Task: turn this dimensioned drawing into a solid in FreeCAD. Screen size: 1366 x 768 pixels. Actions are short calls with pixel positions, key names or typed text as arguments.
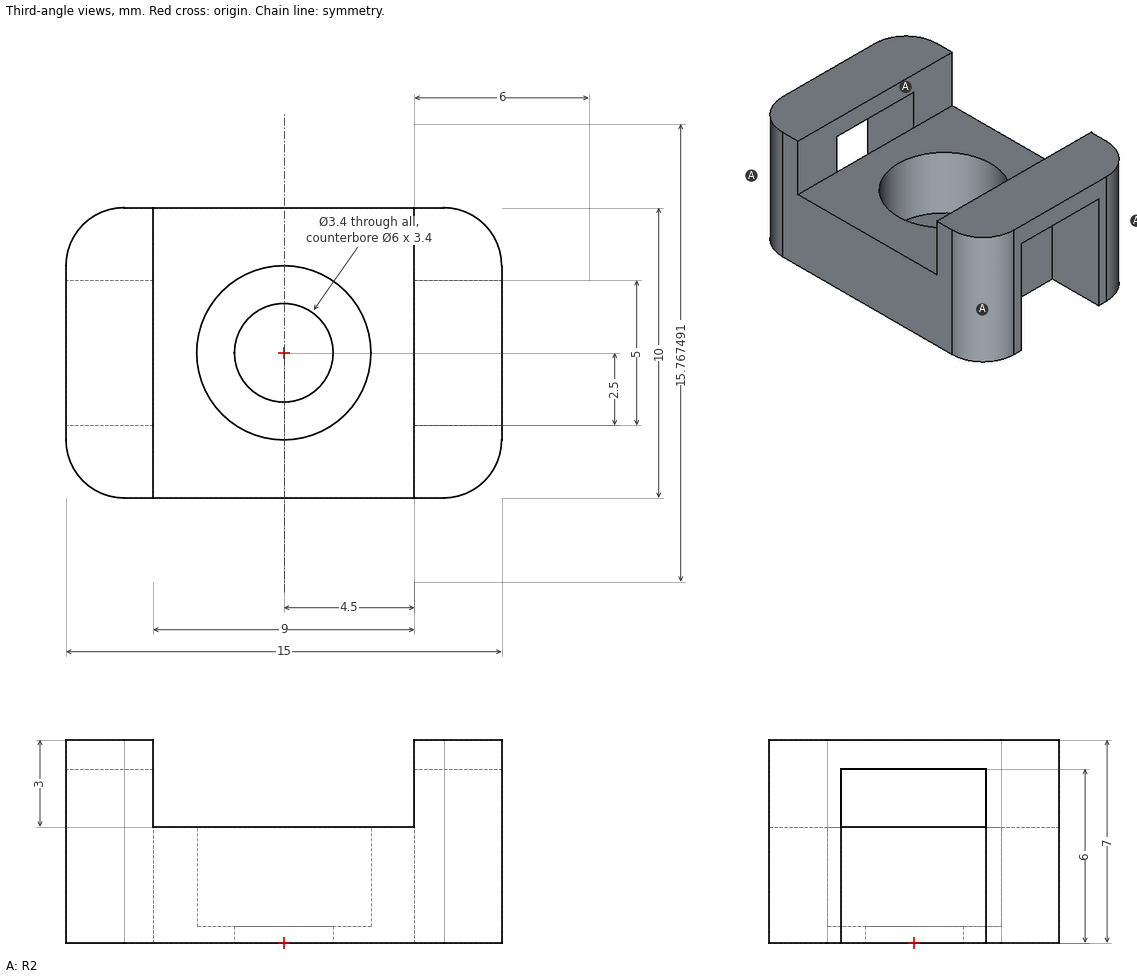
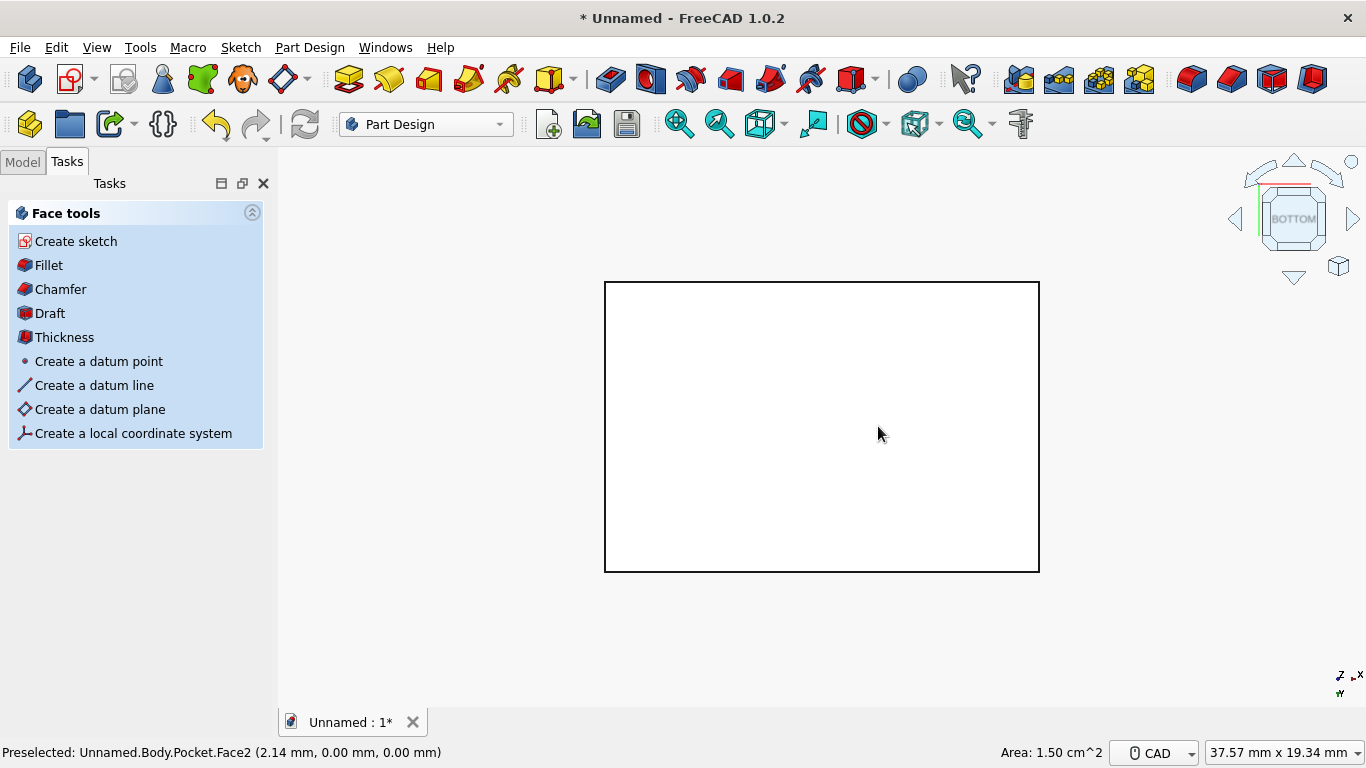
click(70, 80)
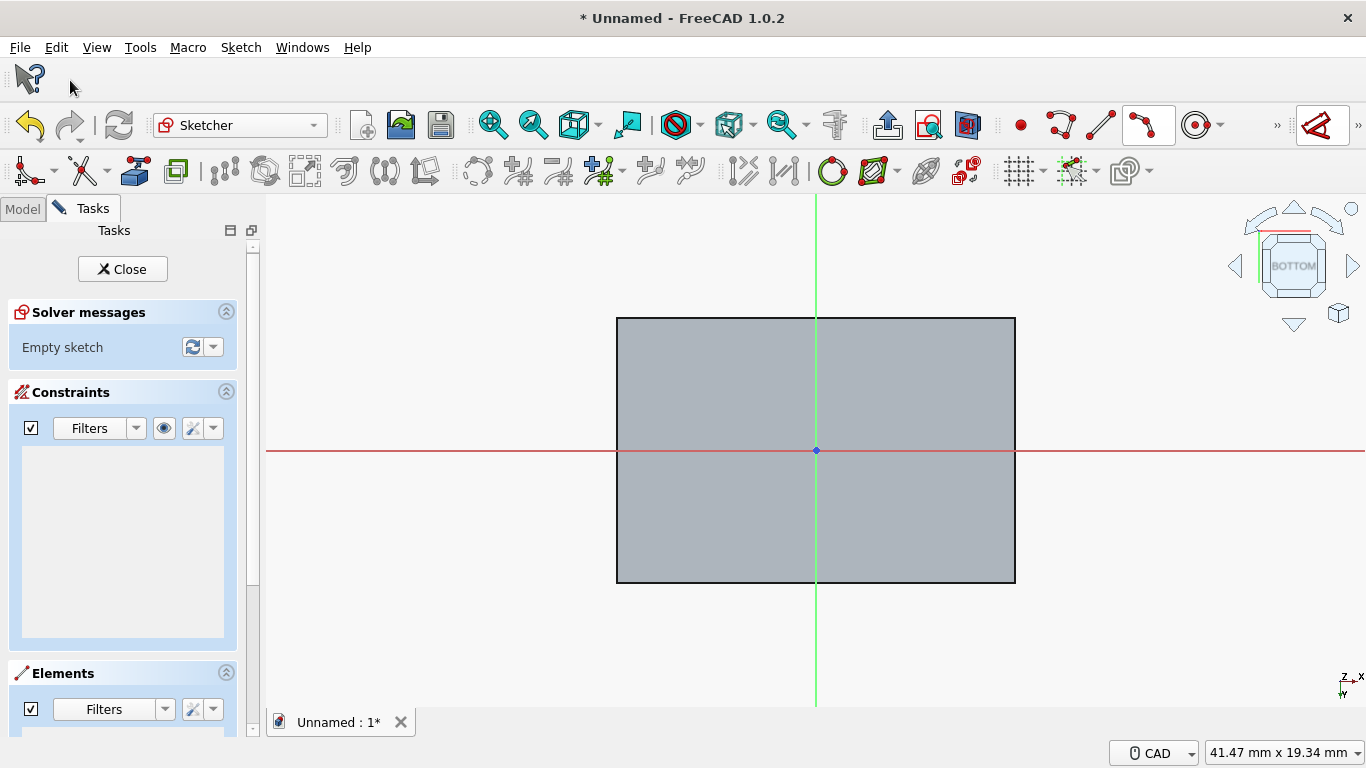
key(g)
key(r)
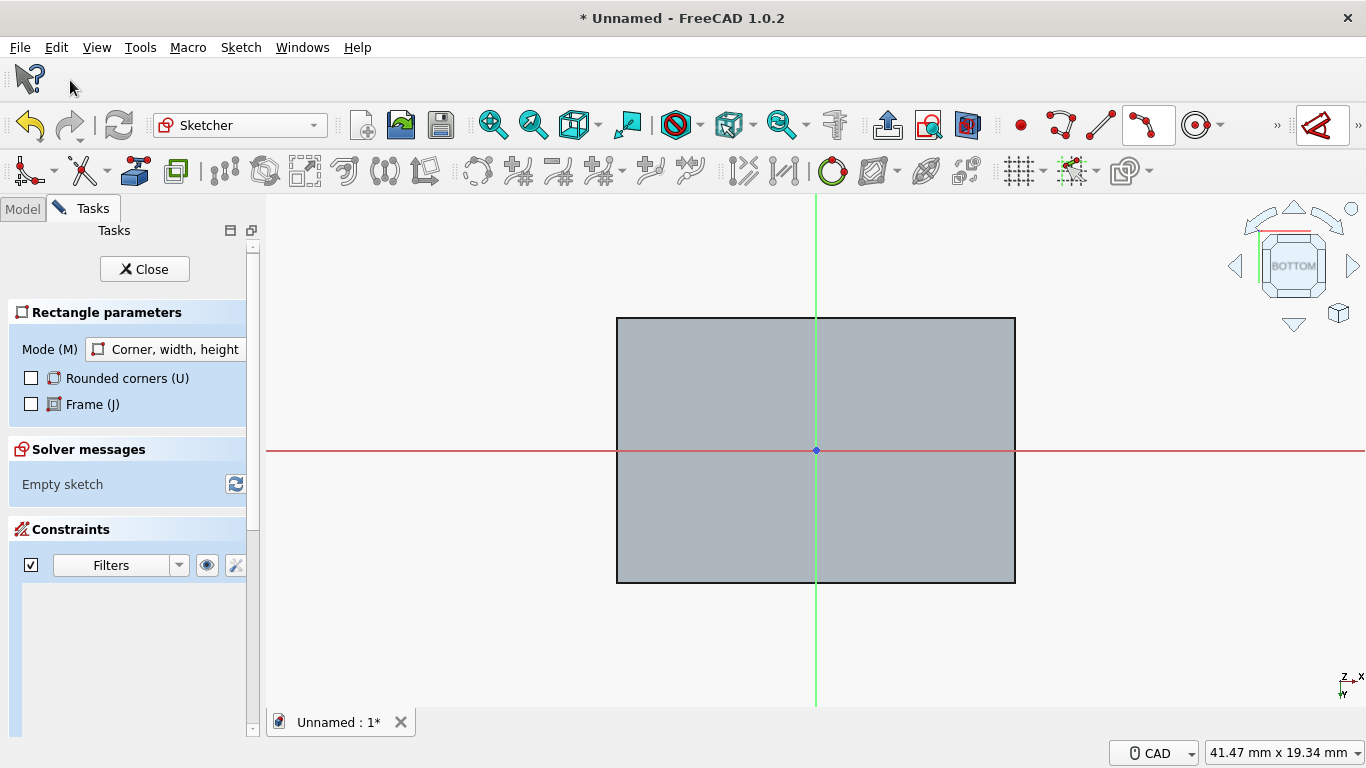
click(935, 384)
click(1095, 517)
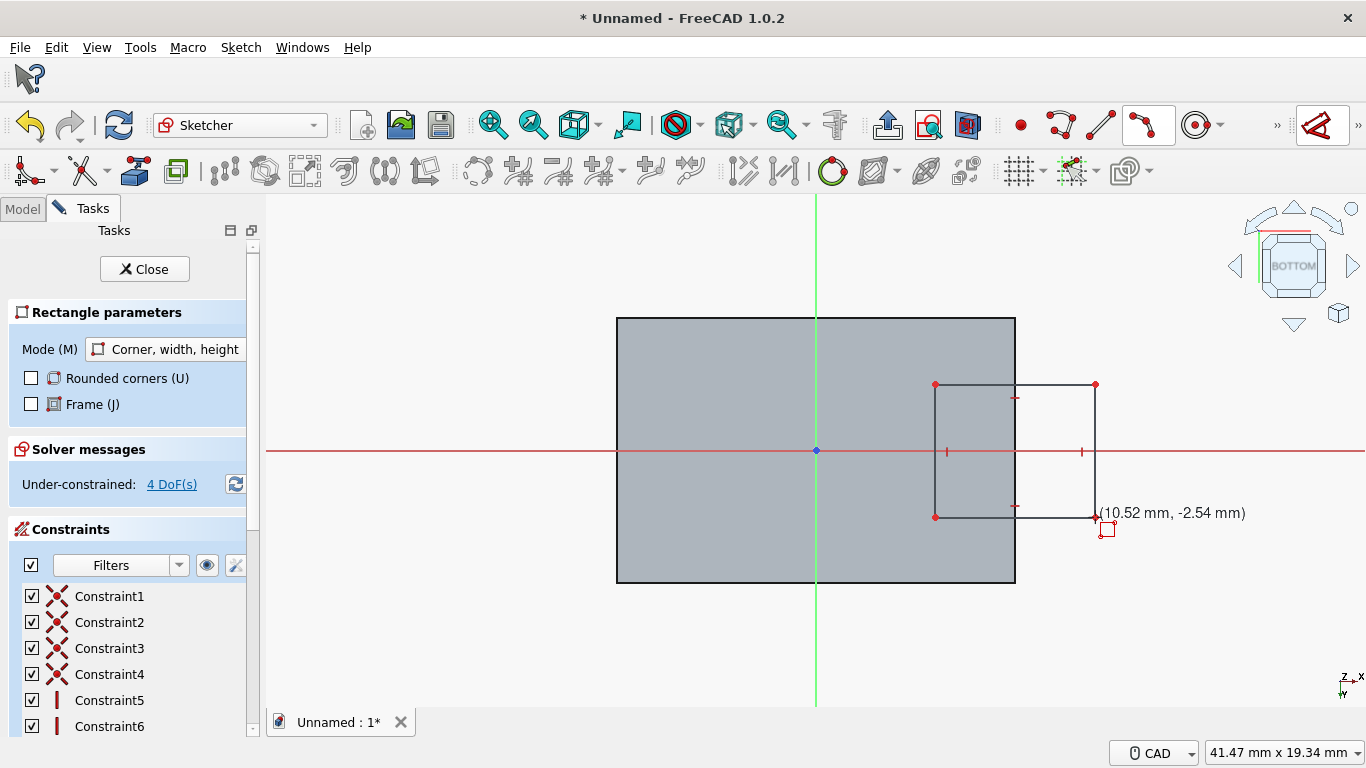
click(537, 384)
click(697, 517)
key(Escape)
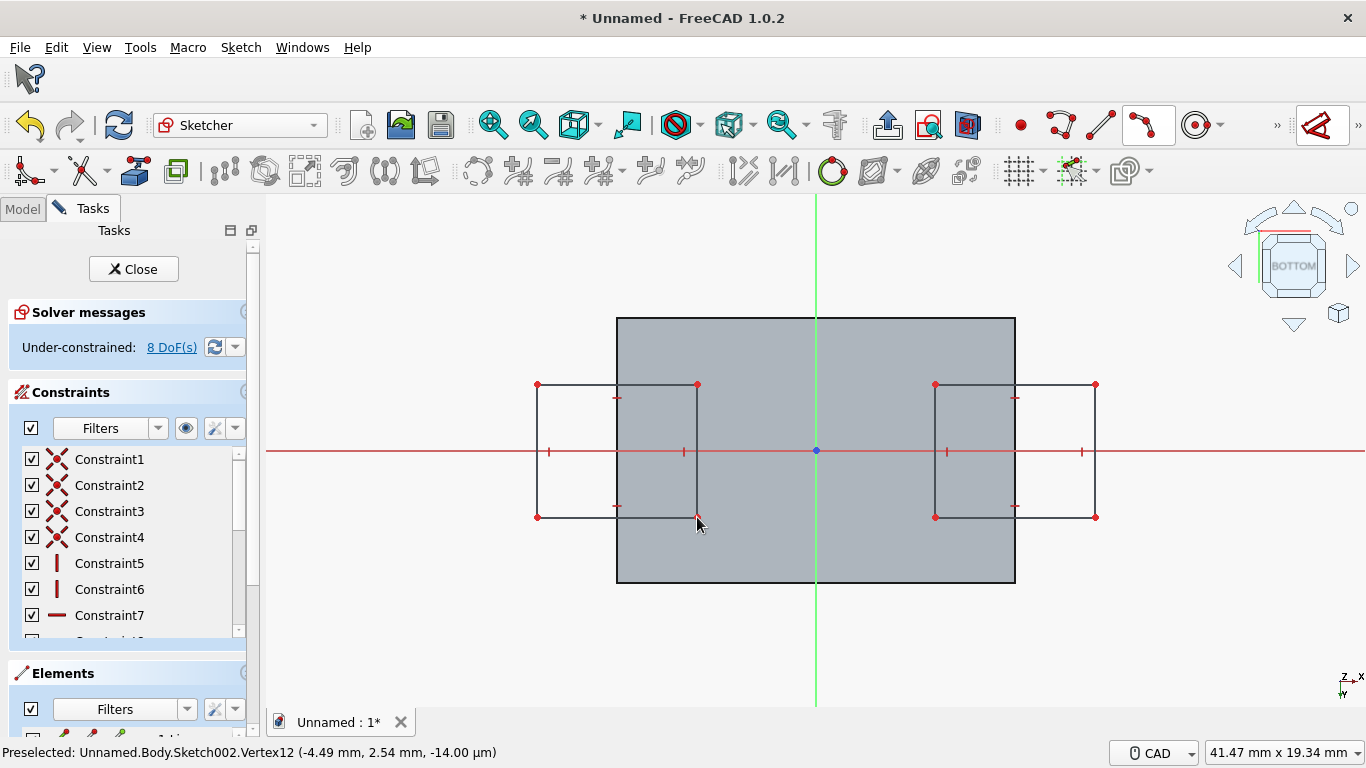
click(1095, 385)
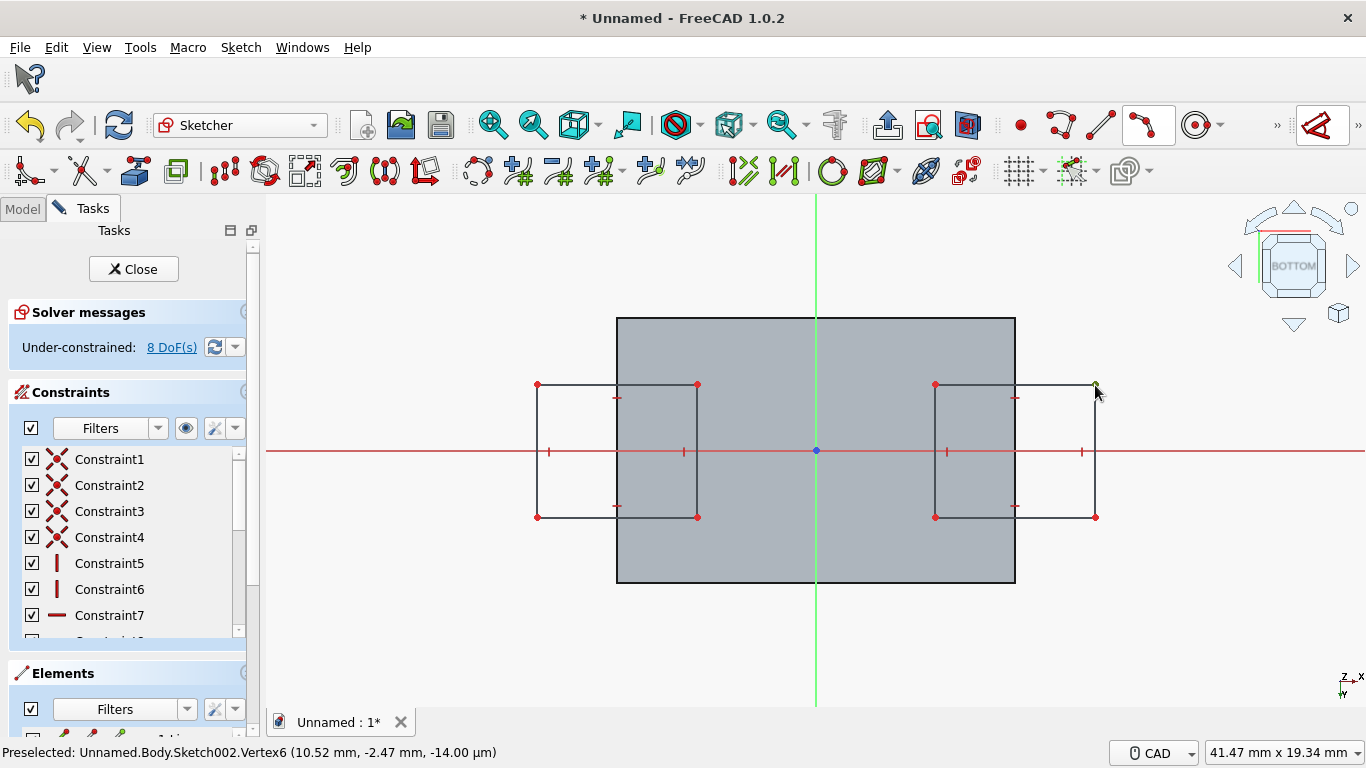
click(537, 385)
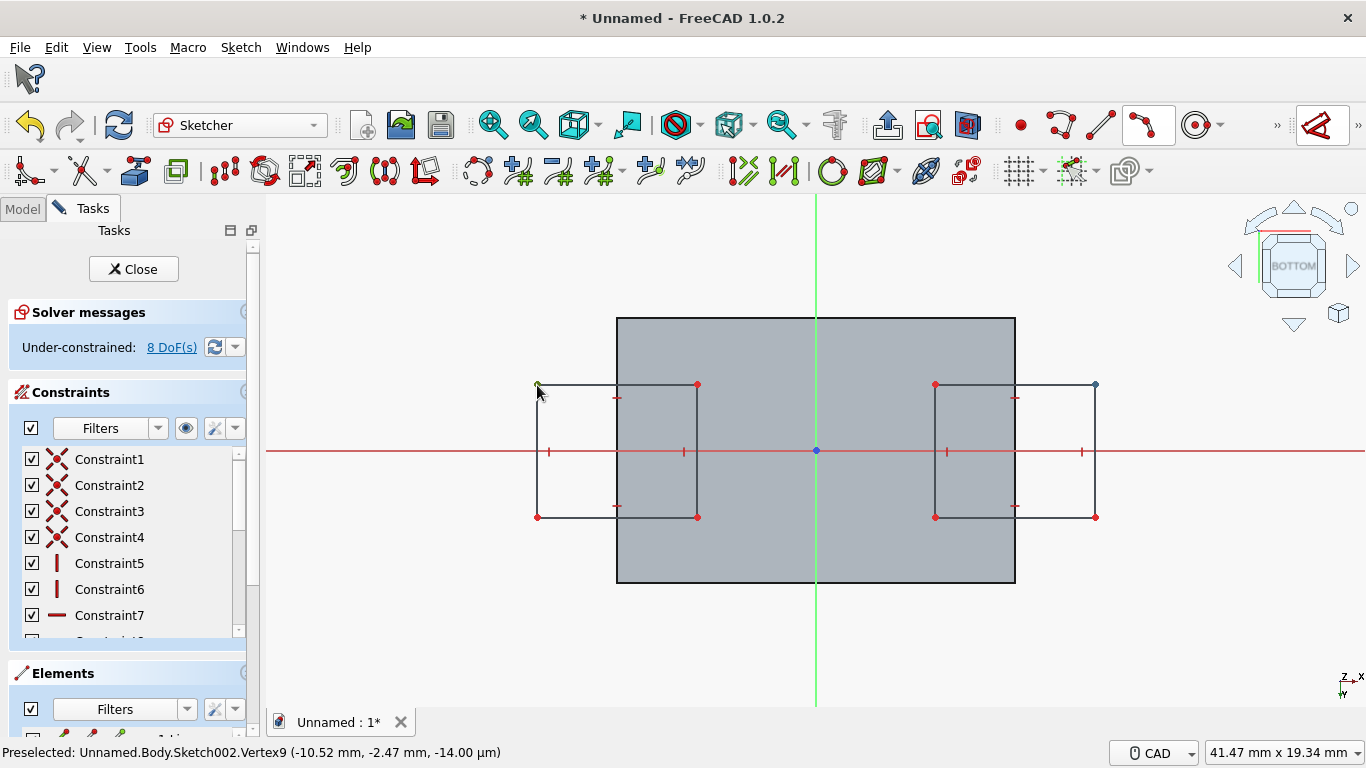
click(816, 646)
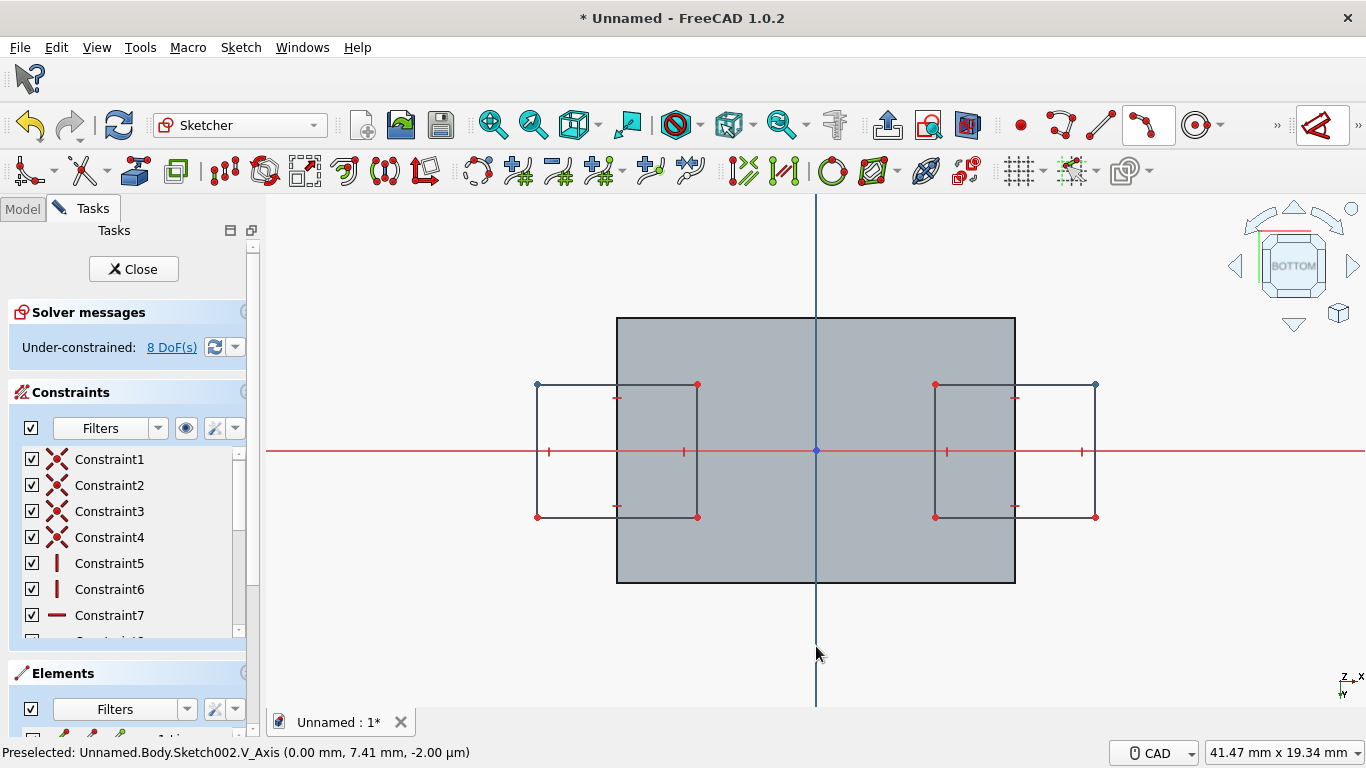
key(s)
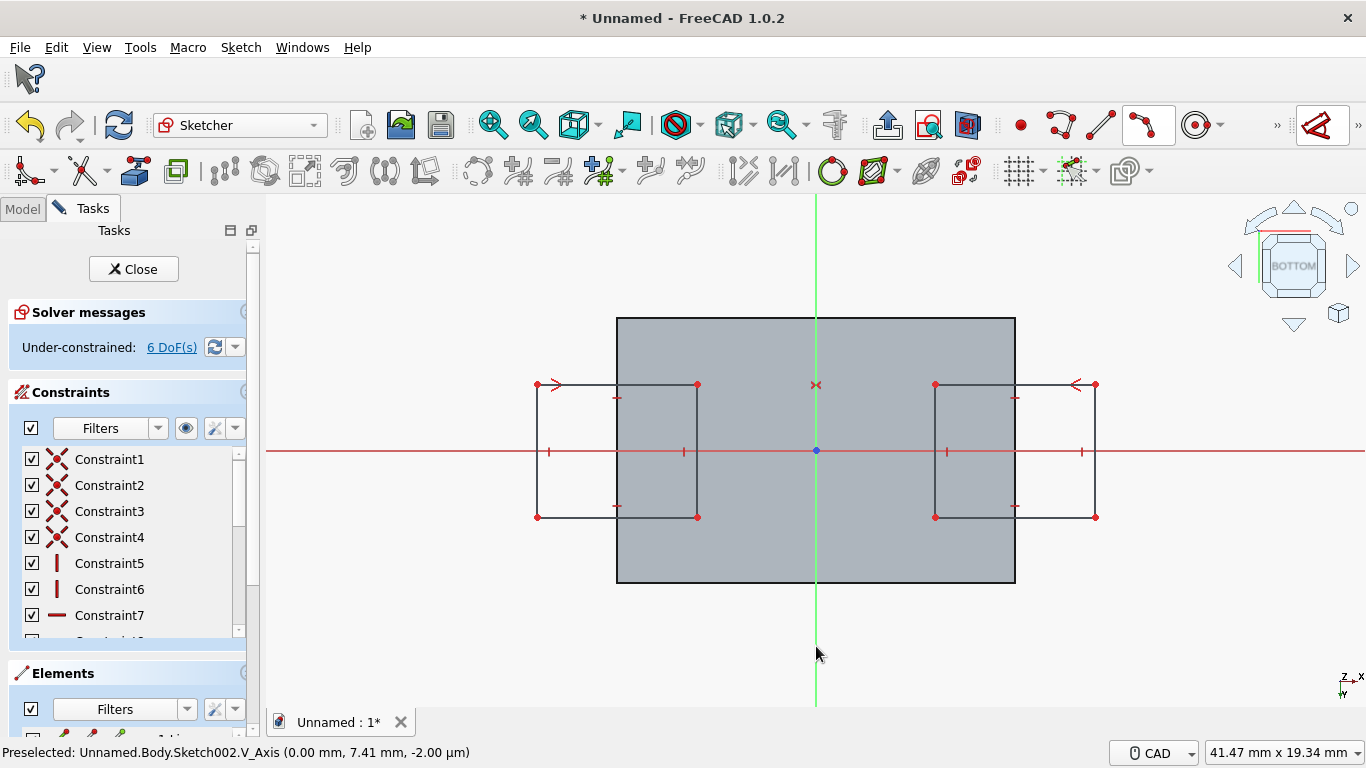
click(935, 518)